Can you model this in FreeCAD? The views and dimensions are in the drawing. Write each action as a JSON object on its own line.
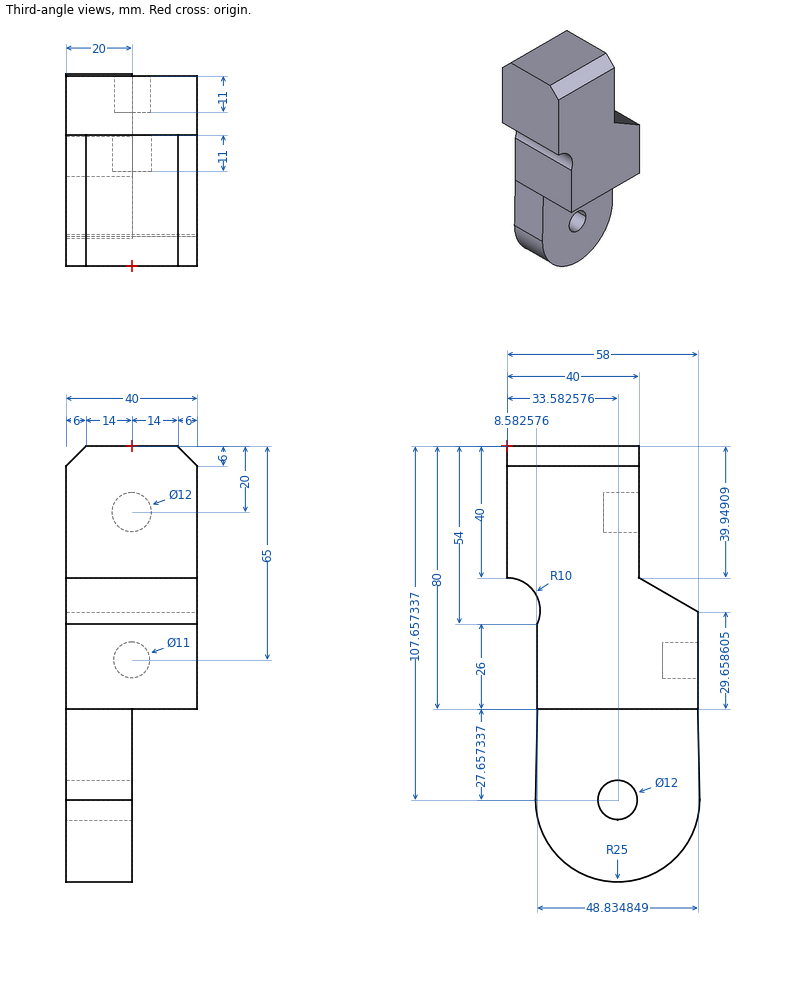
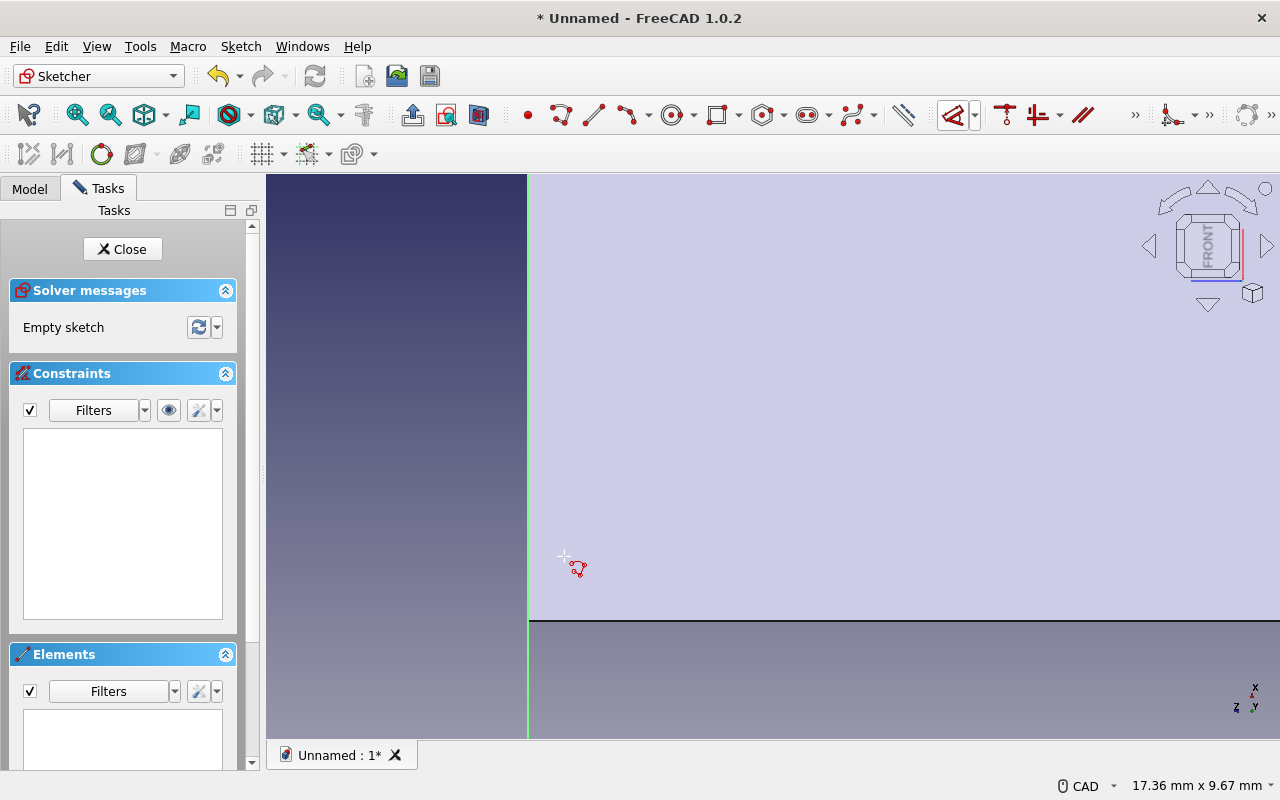
{"action": "left_click", "coordinate": [528, 270]}
{"action": "left_click", "coordinate": [537, 621]}
{"action": "left_click", "coordinate": [878, 621]}
{"action": "left_click", "coordinate": [528, 271]}
{"action": "key", "text": "Escape"}
{"action": "key", "text": "Escape"}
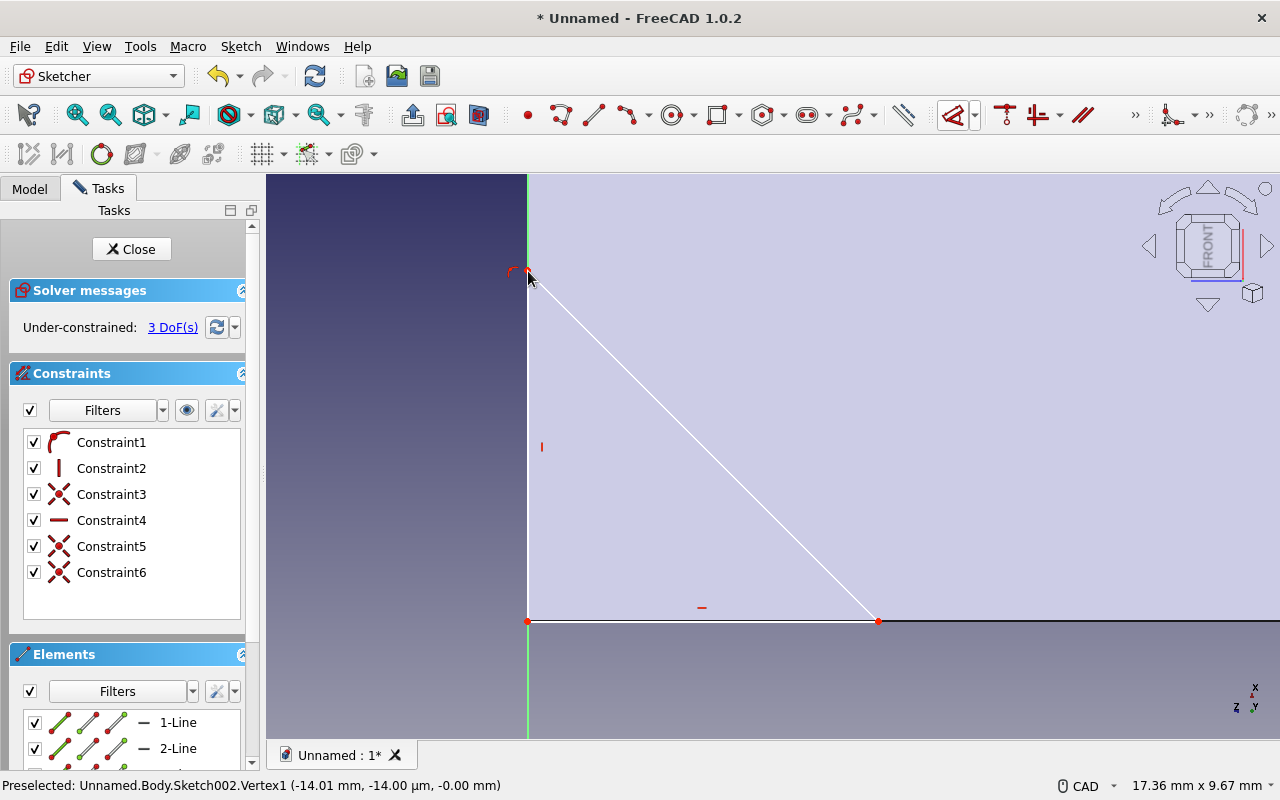
{"action": "left_click", "coordinate": [528, 376]}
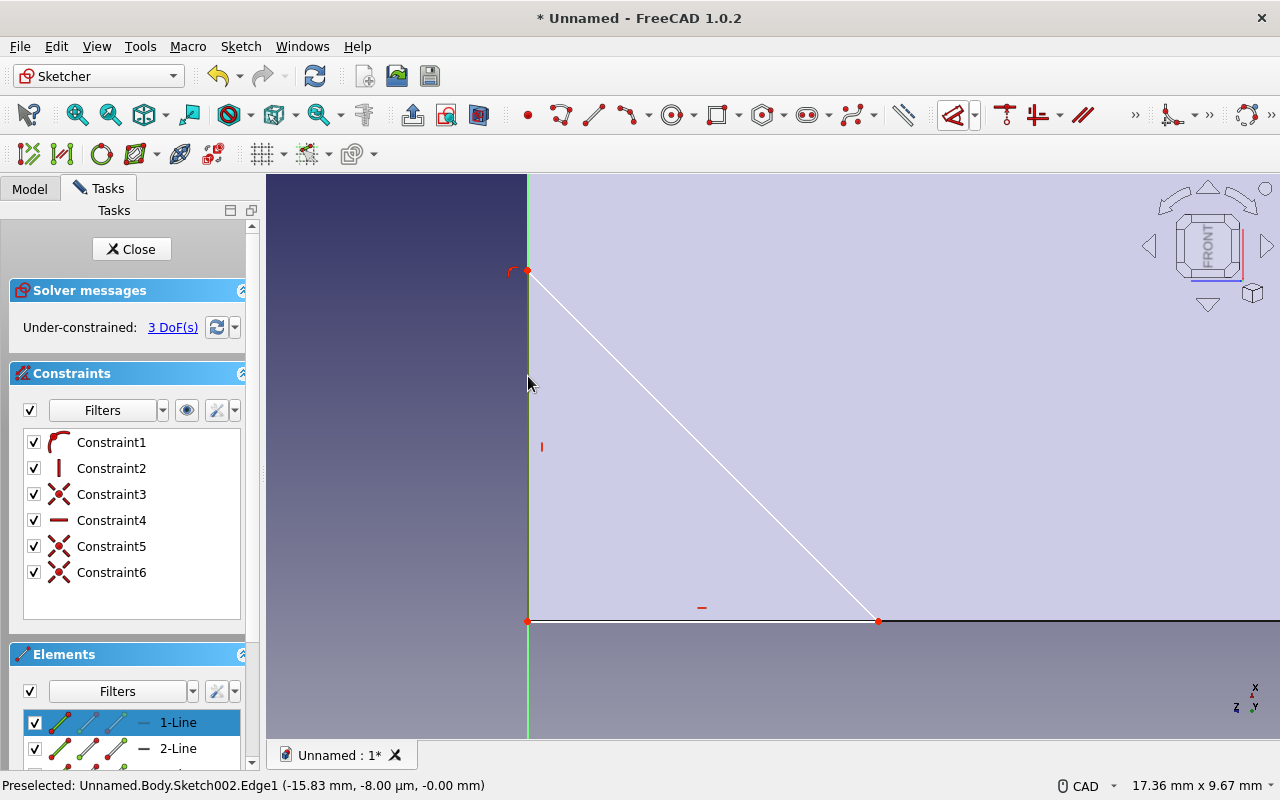
{"action": "key", "text": "i"}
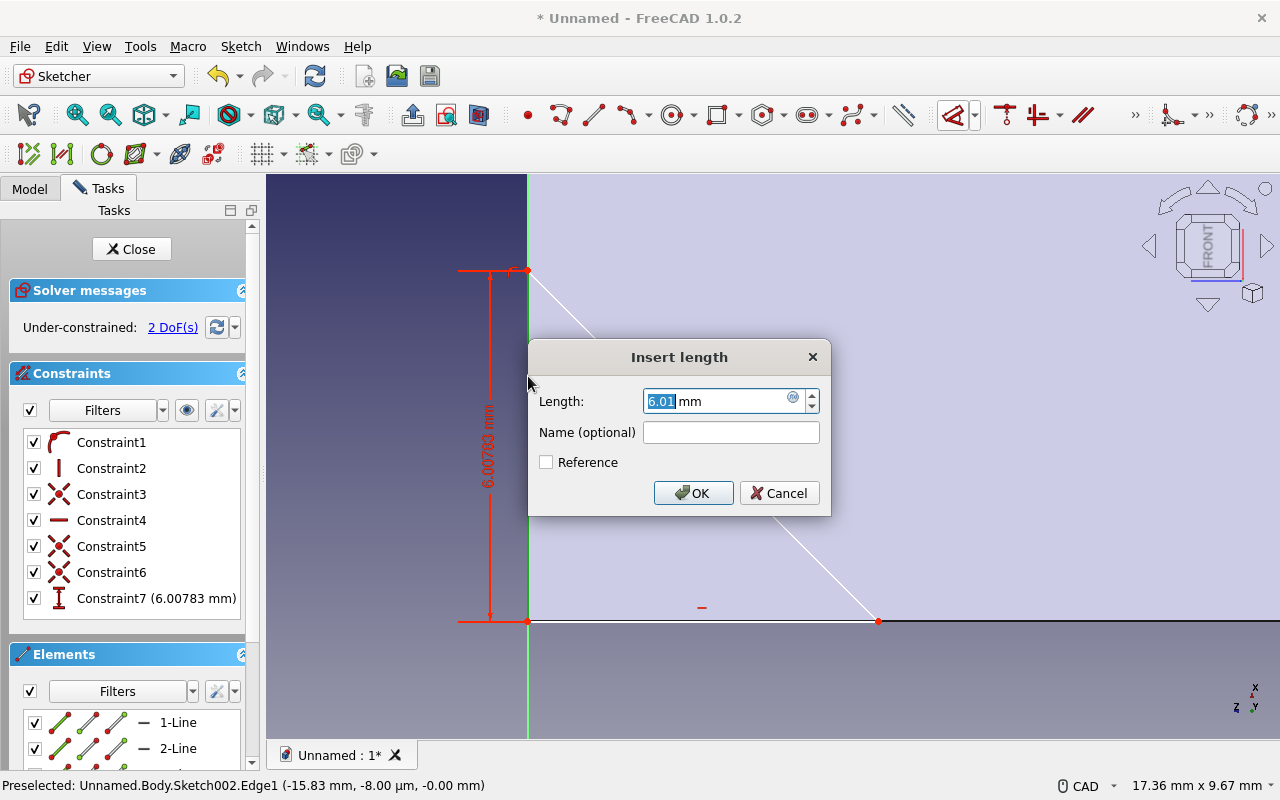
{"action": "type", "text": "6"}
{"action": "key", "text": "Return"}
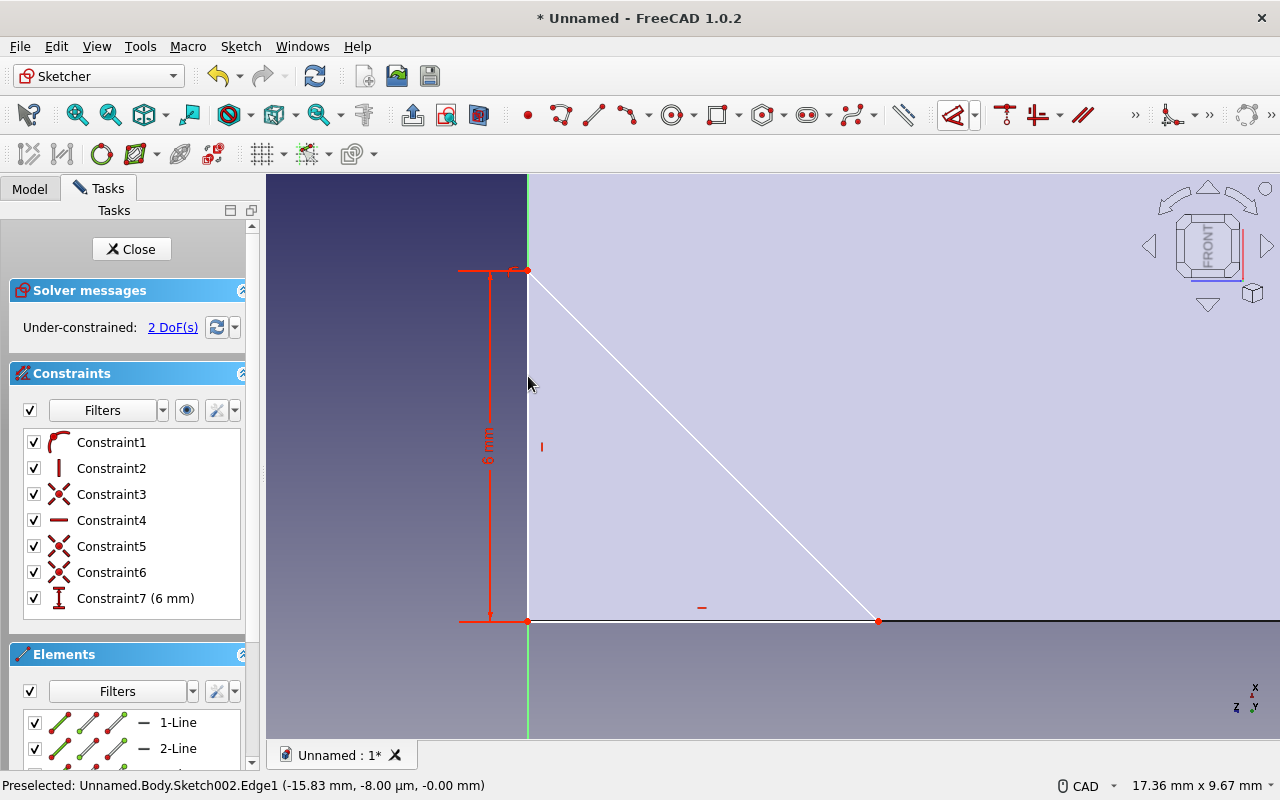
{"action": "left_click", "coordinate": [633, 622]}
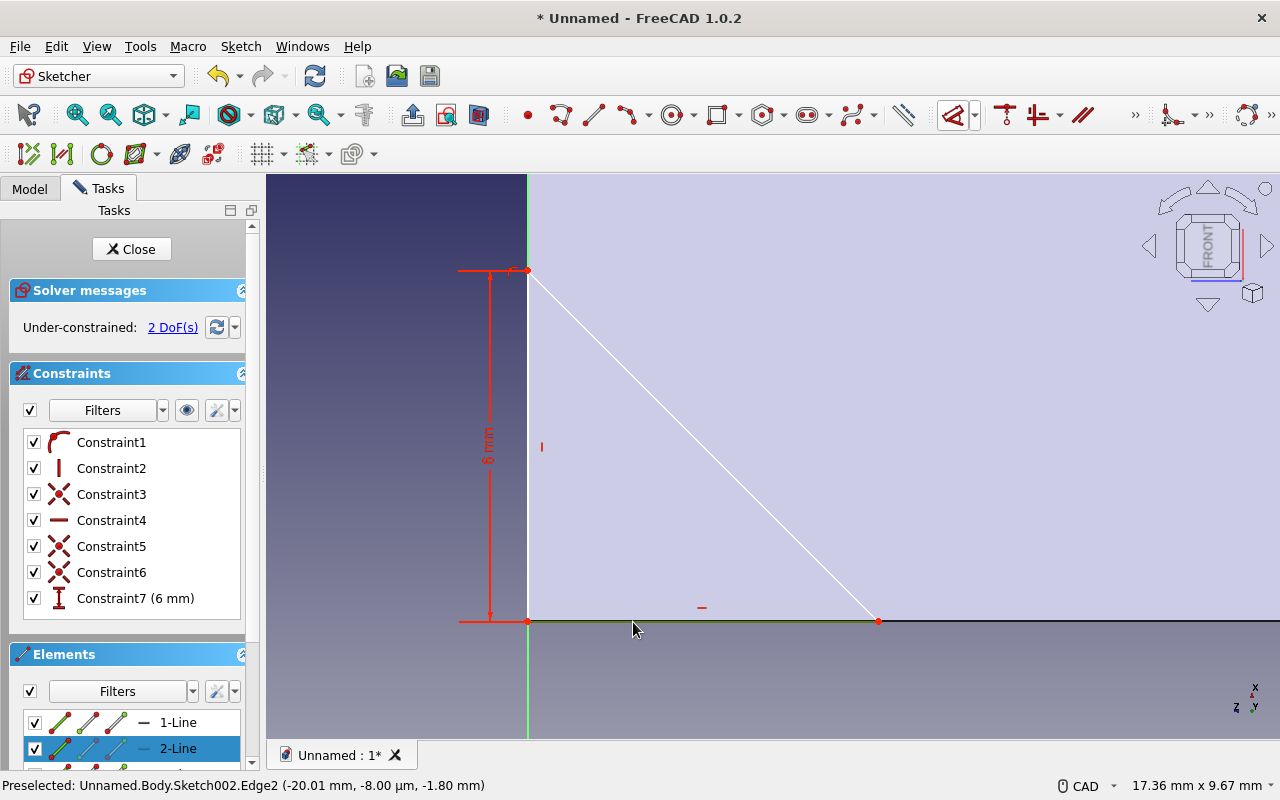
{"action": "key", "text": "l"}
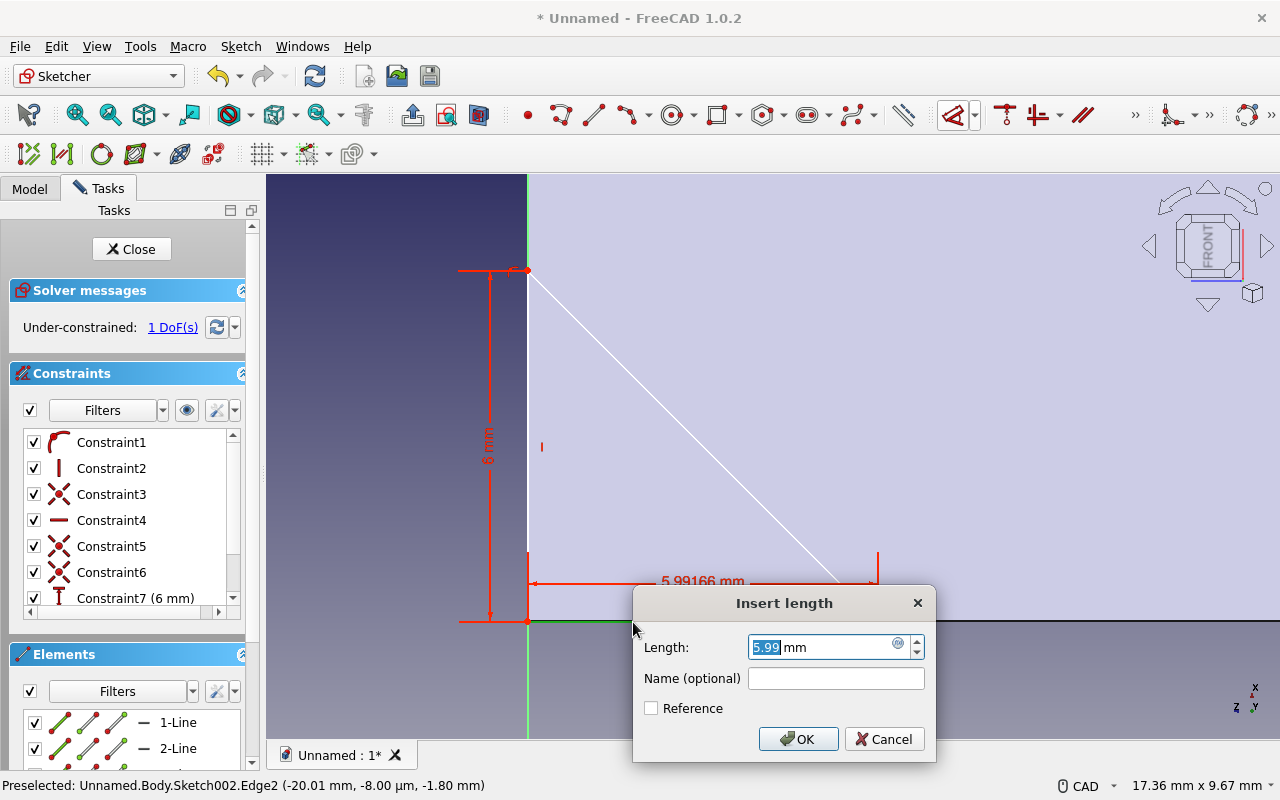
{"action": "type", "text": "6"}
{"action": "key", "text": "Return"}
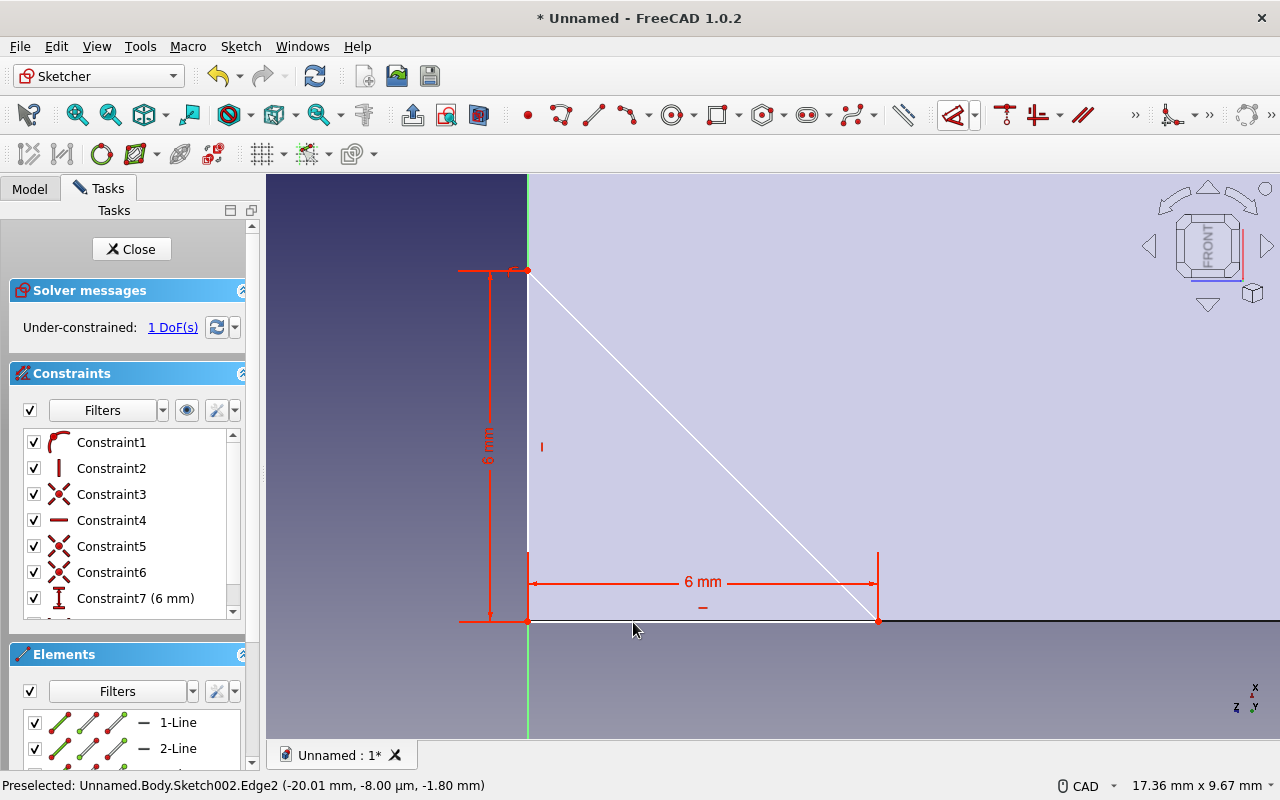
{"action": "left_click", "coordinate": [528, 271]}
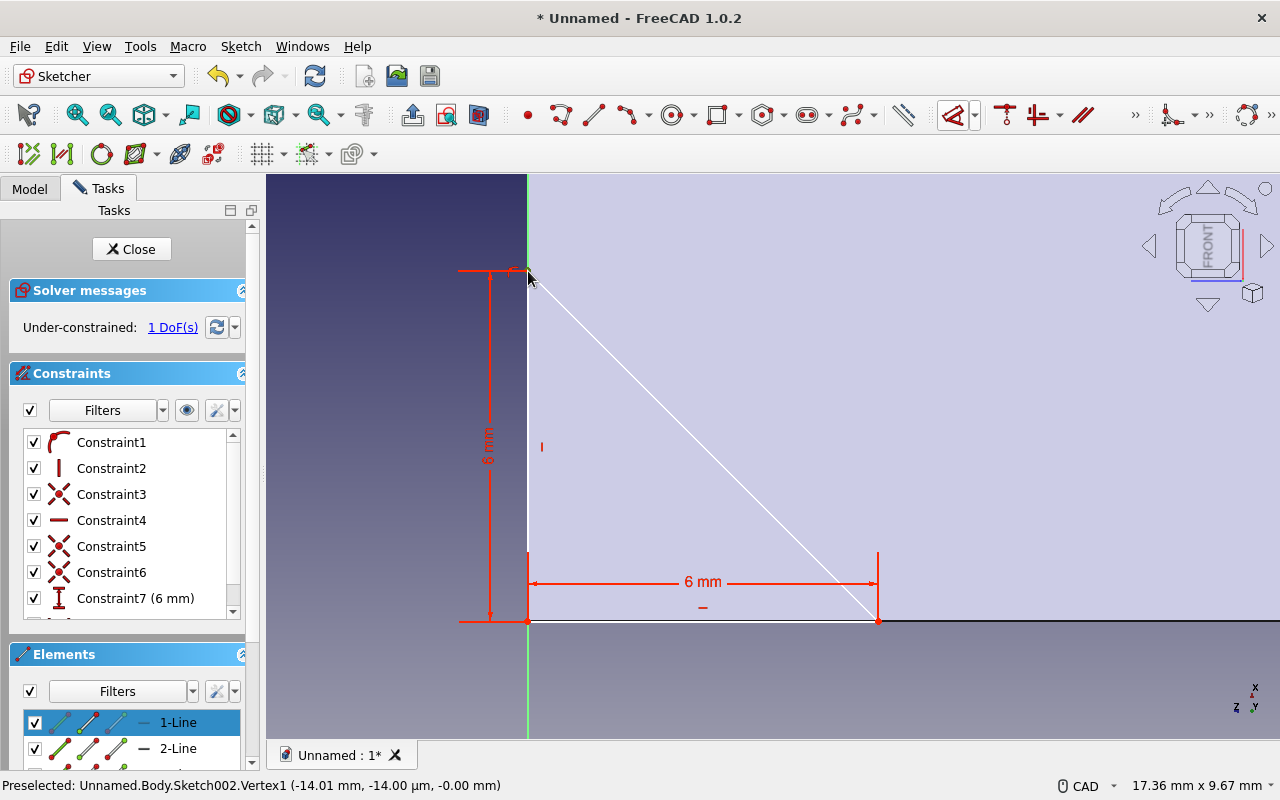
{"action": "key", "text": "i"}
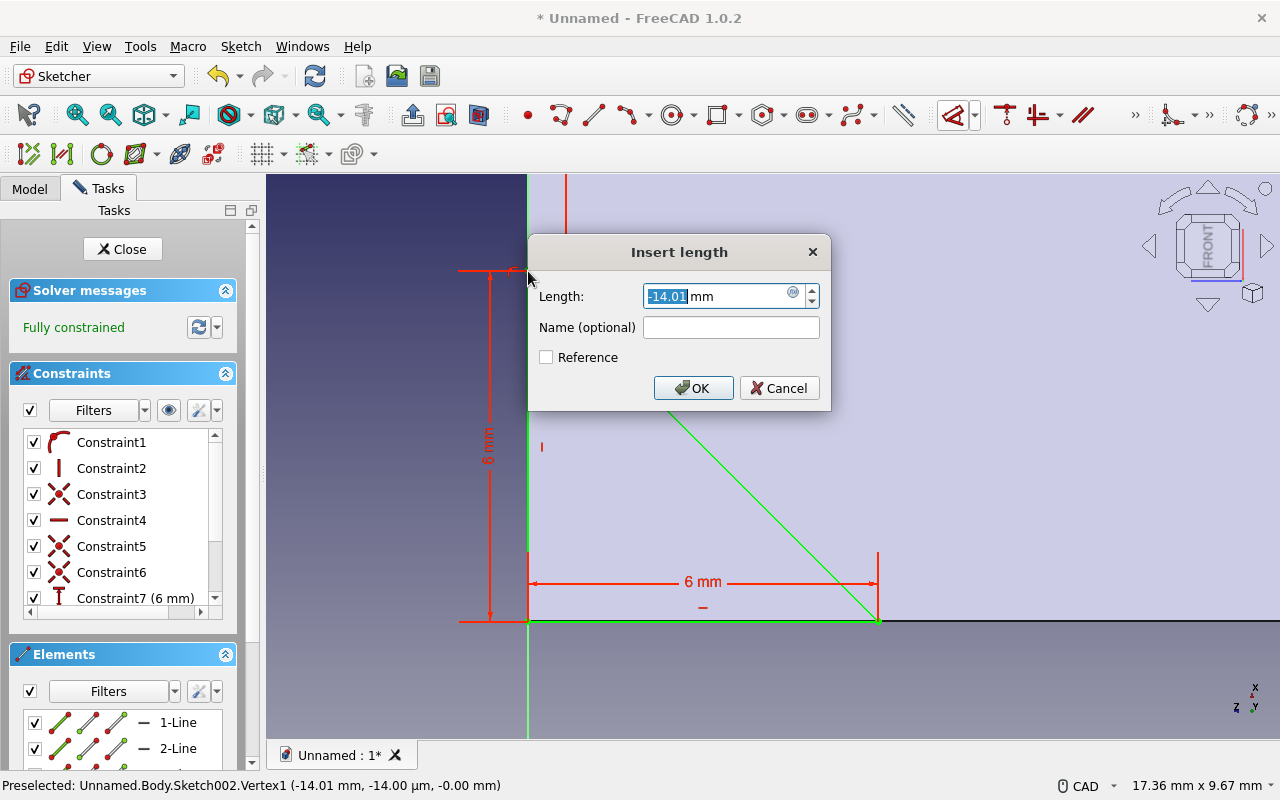
{"action": "type", "text": "-14"}
{"action": "key", "text": "Return"}